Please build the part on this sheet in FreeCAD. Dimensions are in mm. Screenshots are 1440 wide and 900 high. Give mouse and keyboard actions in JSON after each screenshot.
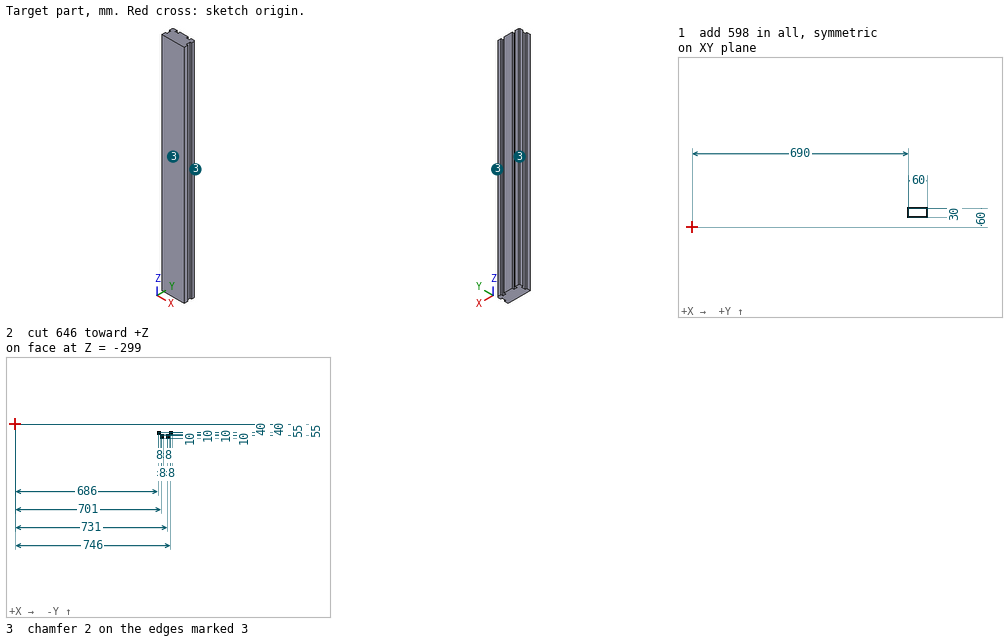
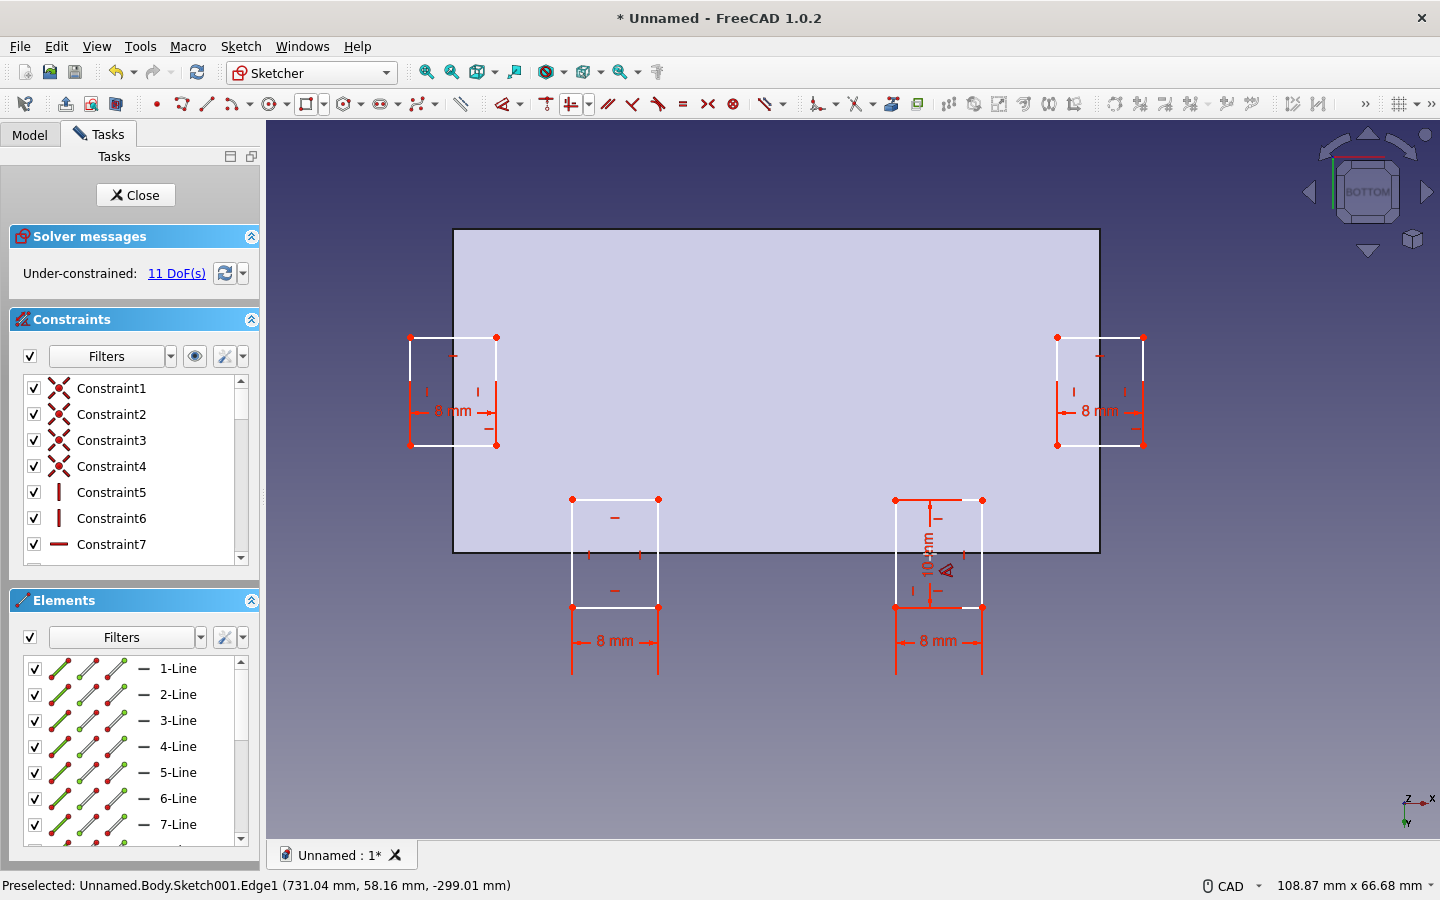
{"action": "left_click", "coordinate": [1057, 370]}
{"action": "left_click", "coordinate": [1091, 392]}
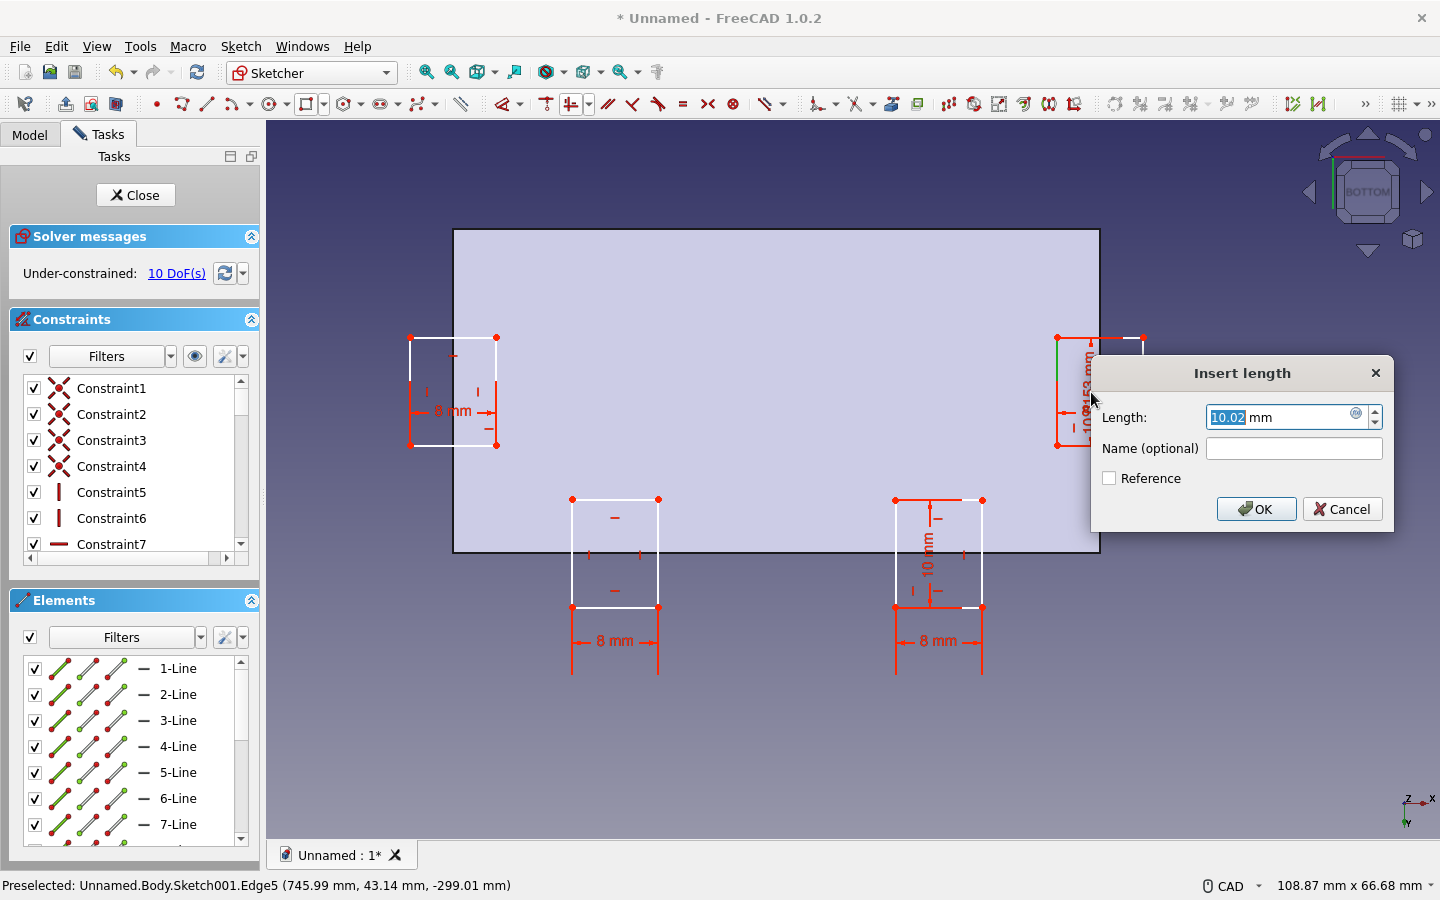
{"action": "type", "text": "10"}
{"action": "key", "text": "Return"}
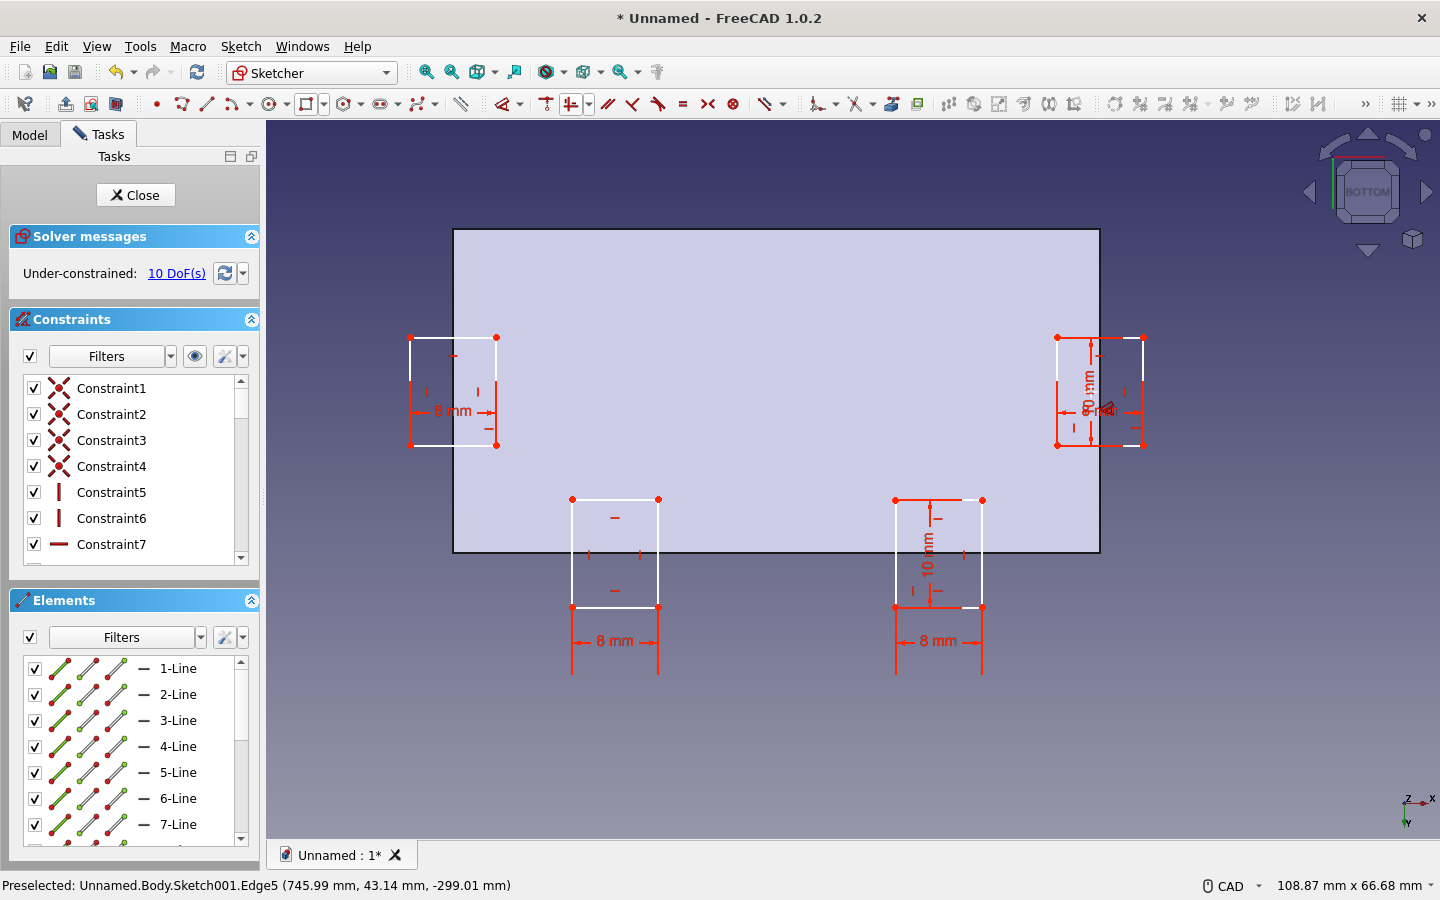
{"action": "left_click", "coordinate": [410, 370]}
{"action": "left_click", "coordinate": [376, 392]}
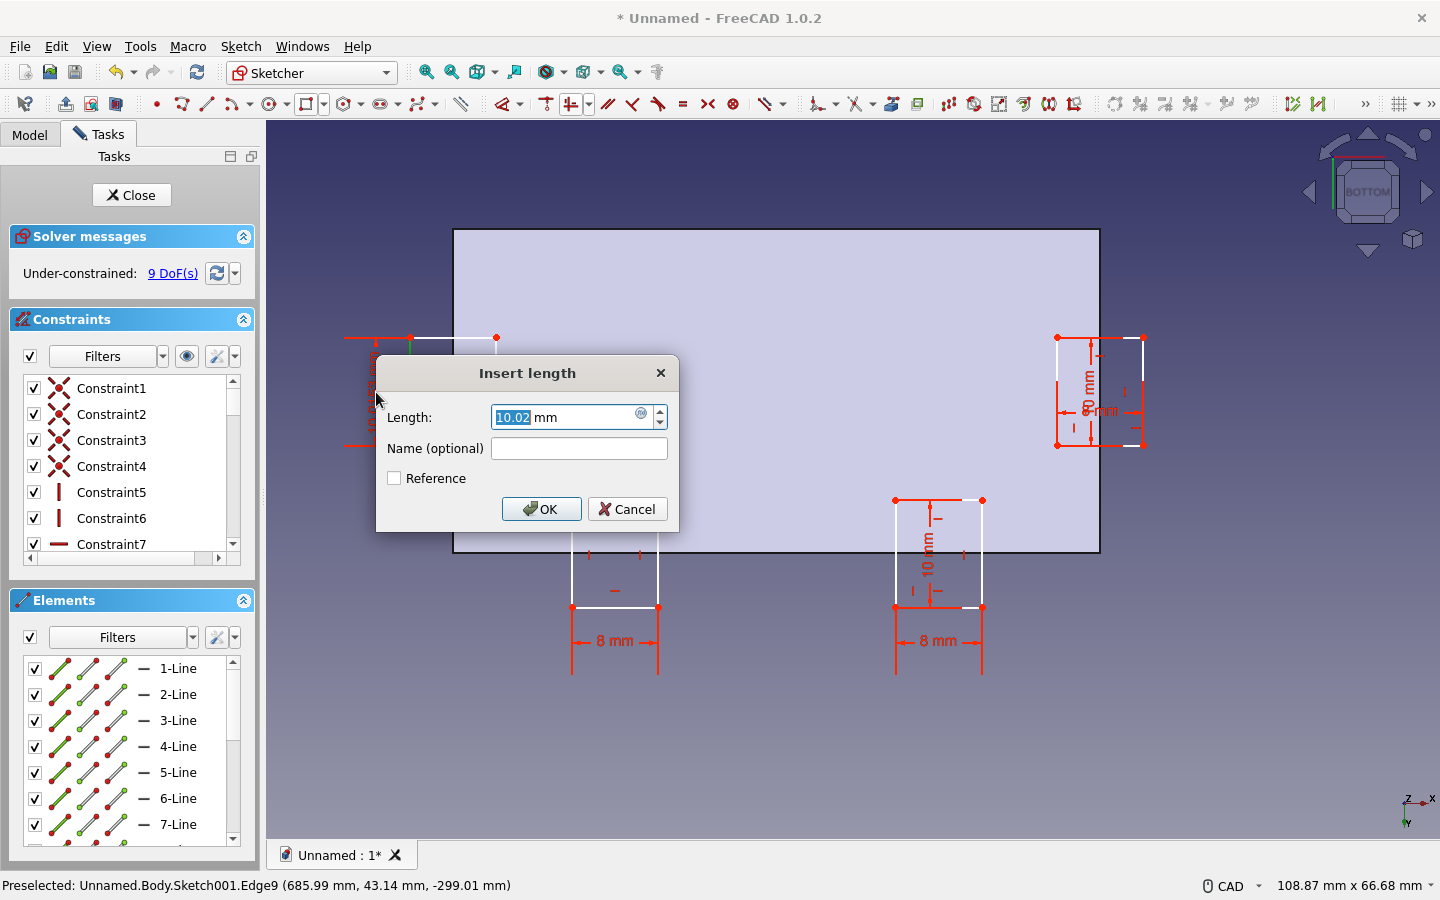
{"action": "type", "text": "10"}
{"action": "key", "text": "Return"}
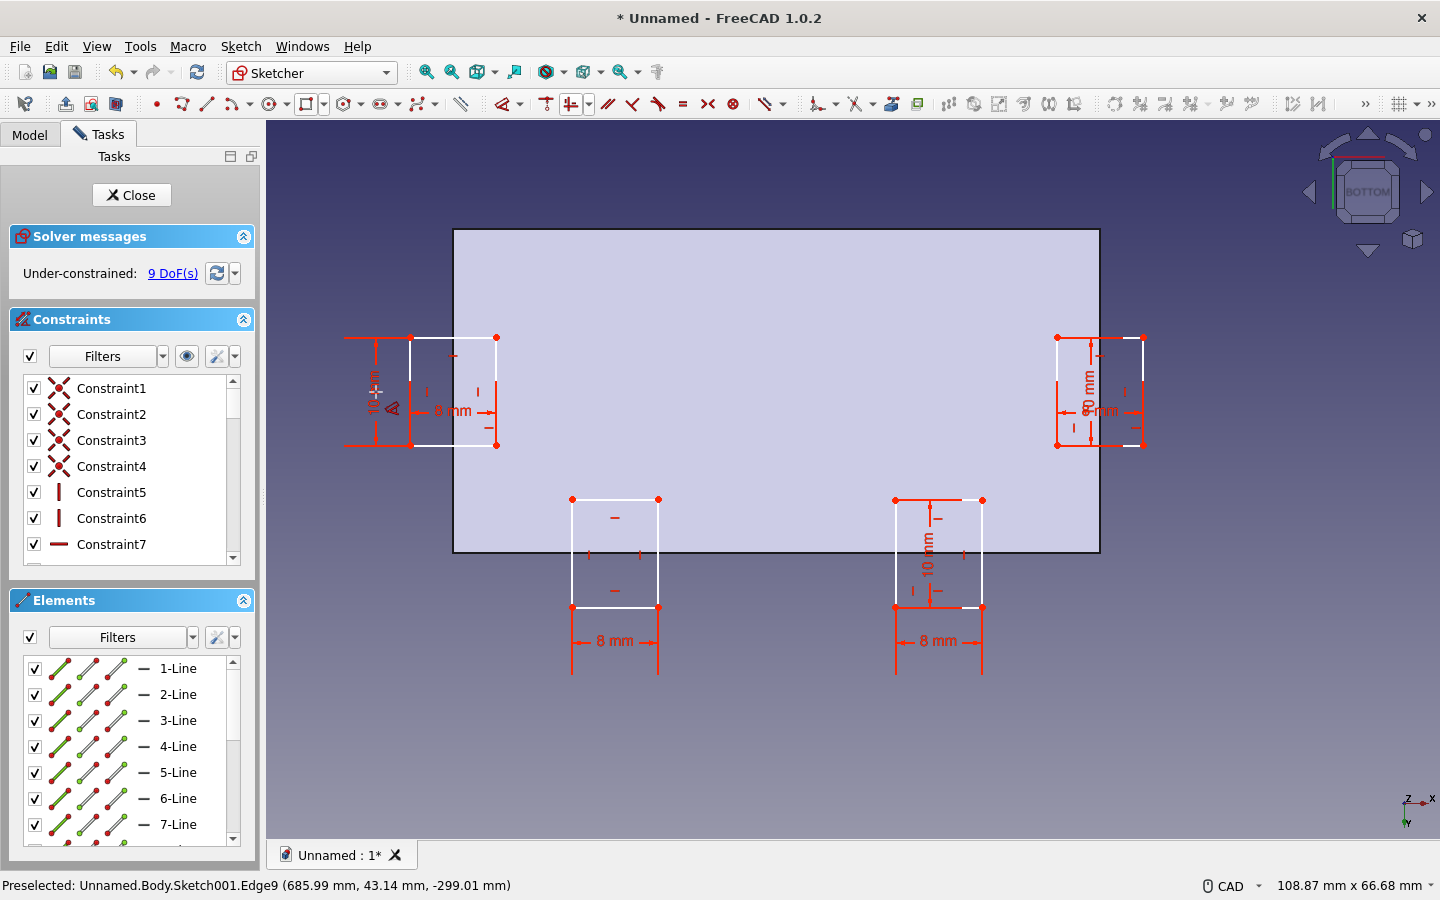
{"action": "left_click", "coordinate": [572, 532]}
{"action": "left_click", "coordinate": [538, 554]}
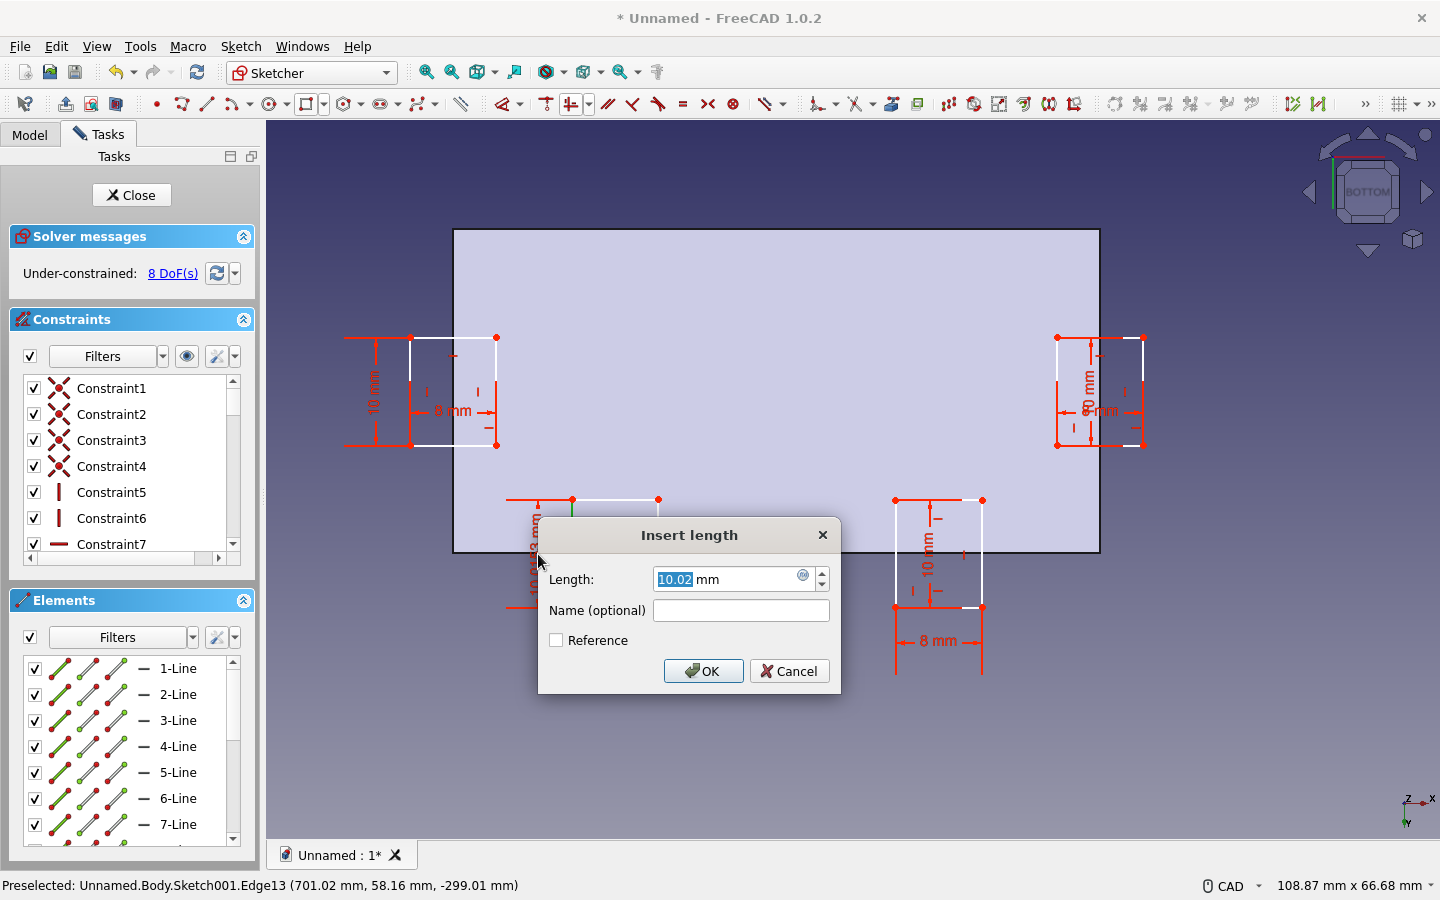
{"action": "type", "text": "10"}
{"action": "key", "text": "Return"}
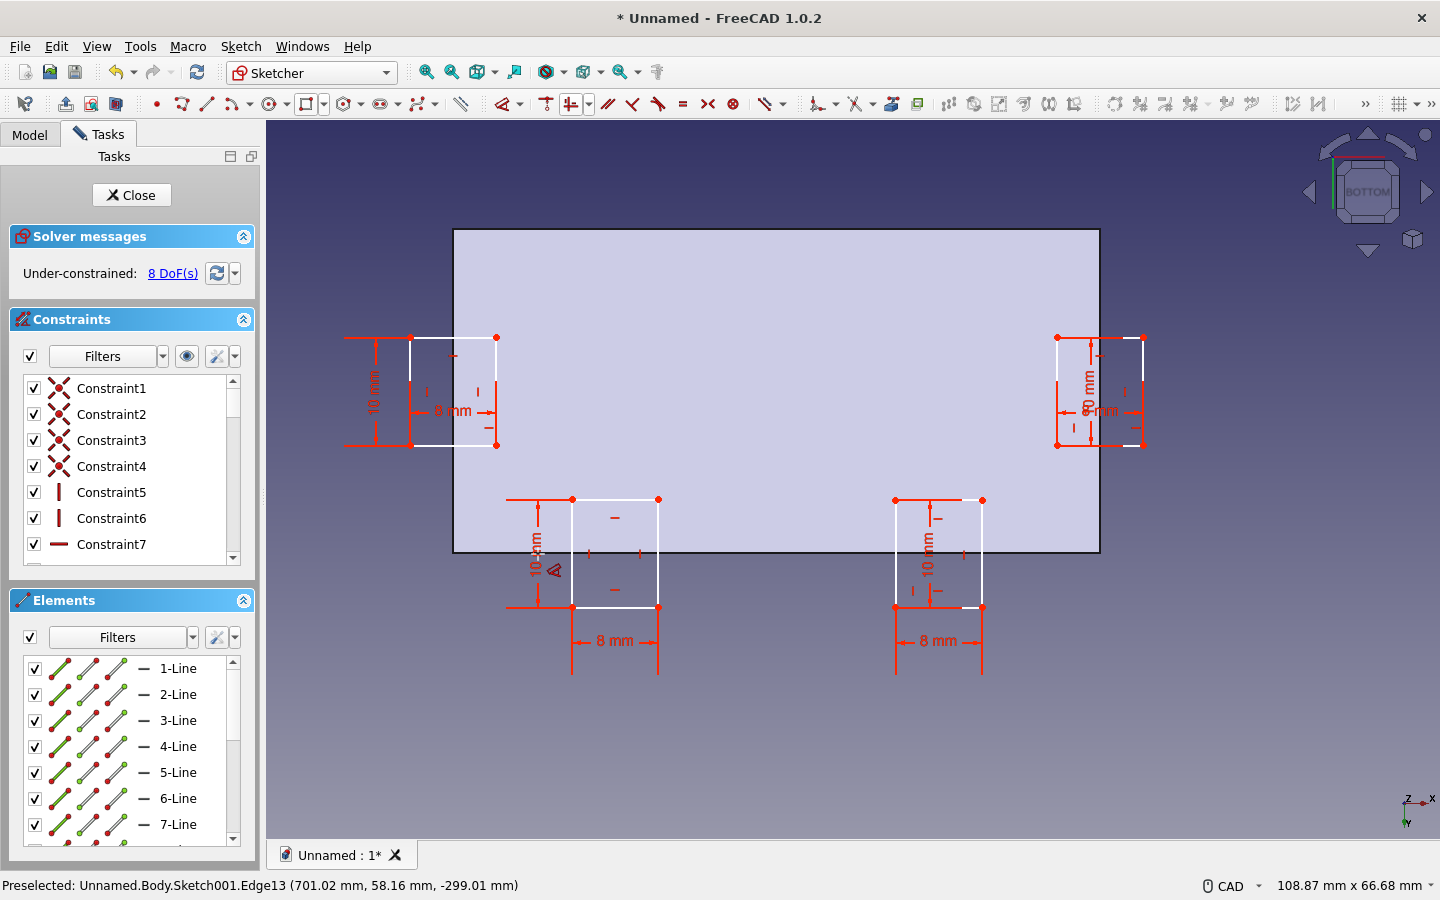
{"action": "left_click", "coordinate": [896, 500]}
{"action": "left_click", "coordinate": [930, 324]}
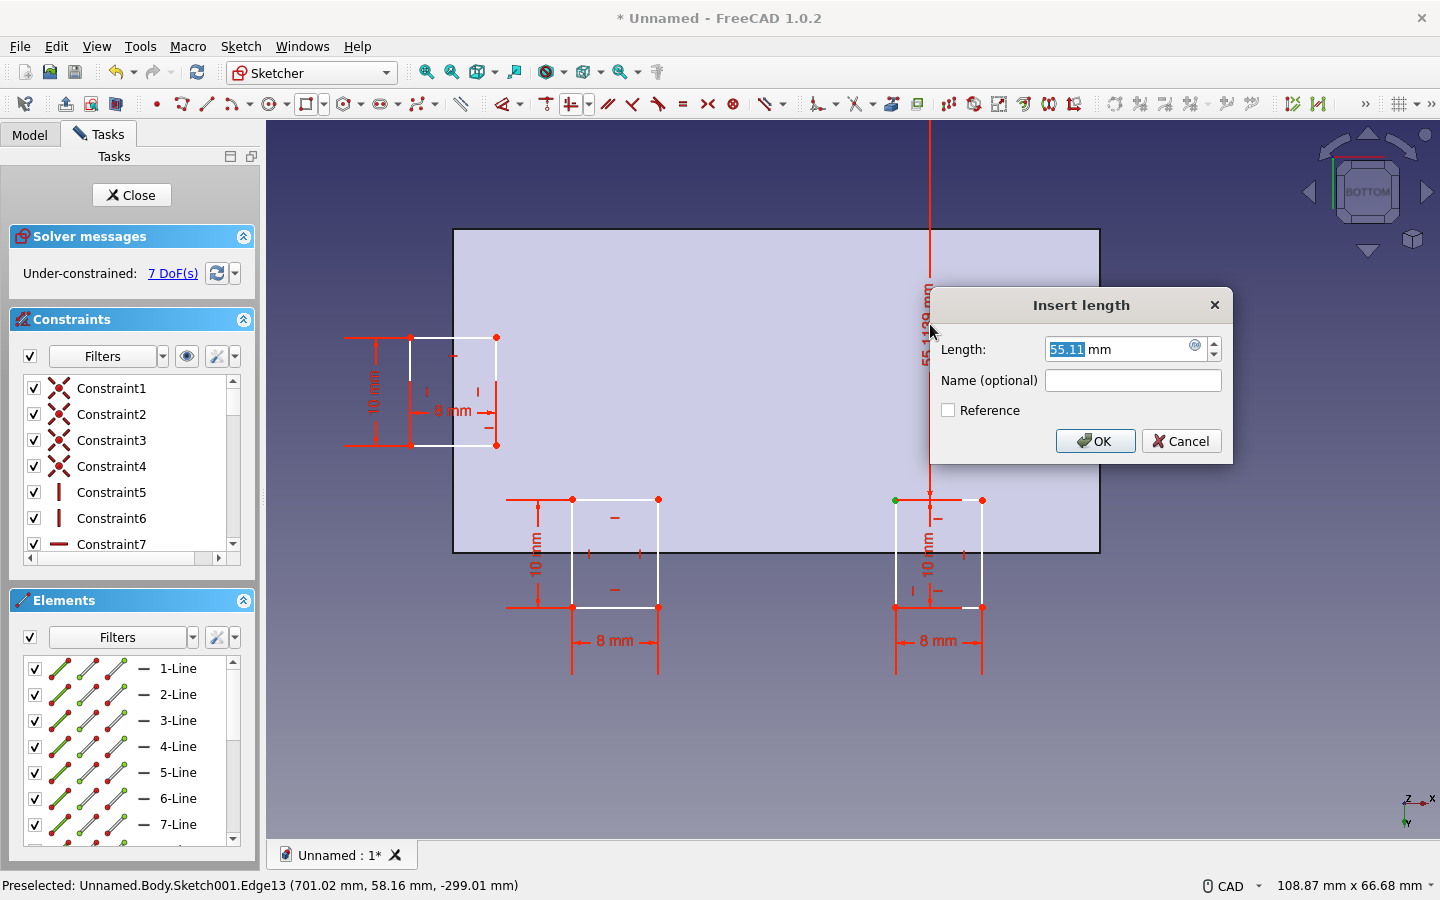
{"action": "type", "text": "55"}
{"action": "key", "text": "Return"}